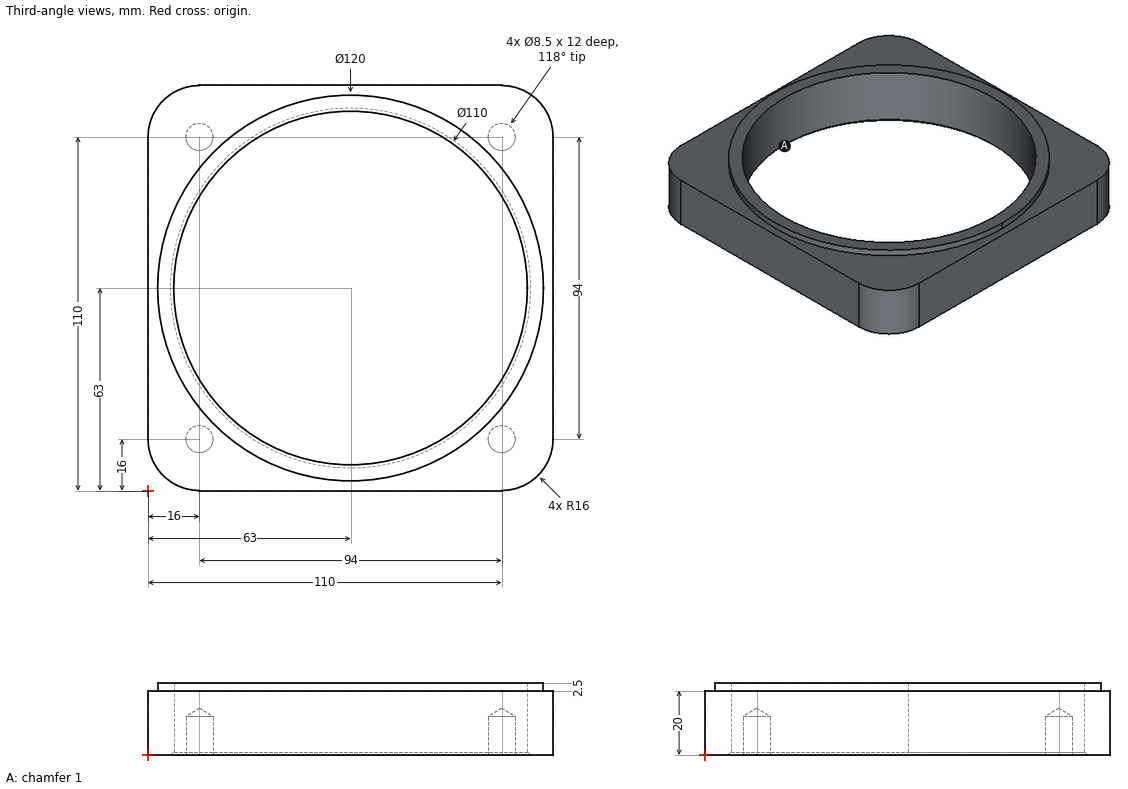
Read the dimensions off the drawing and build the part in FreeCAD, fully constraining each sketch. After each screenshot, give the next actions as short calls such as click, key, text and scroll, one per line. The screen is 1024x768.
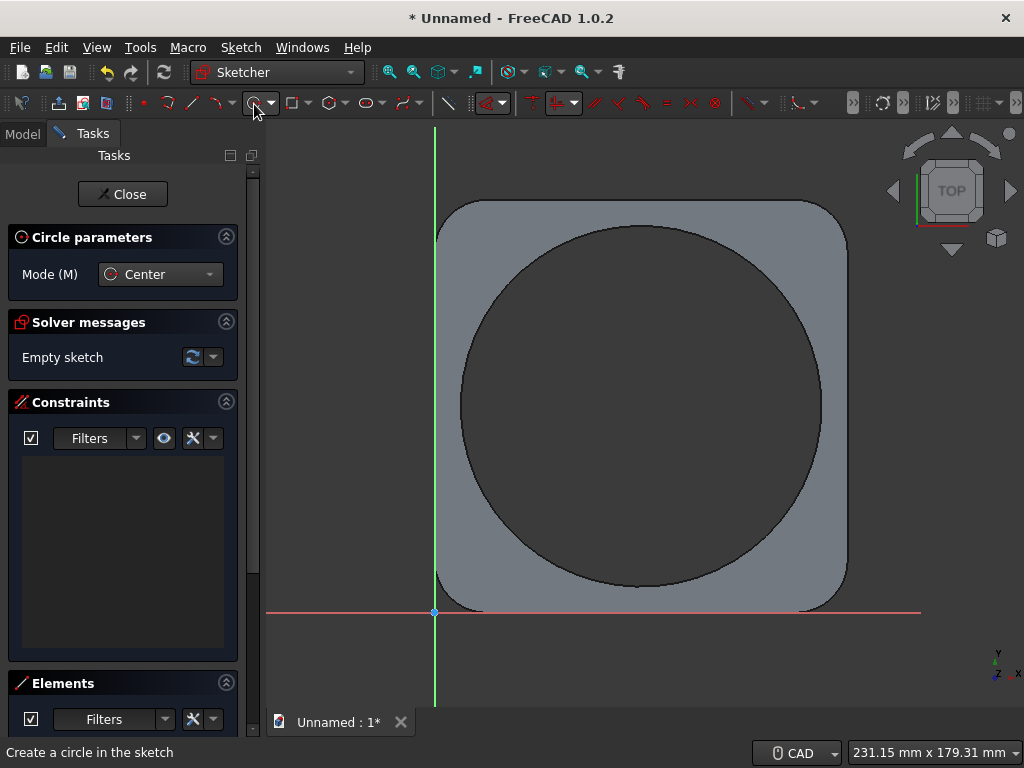
scroll(795, 252, up, 3)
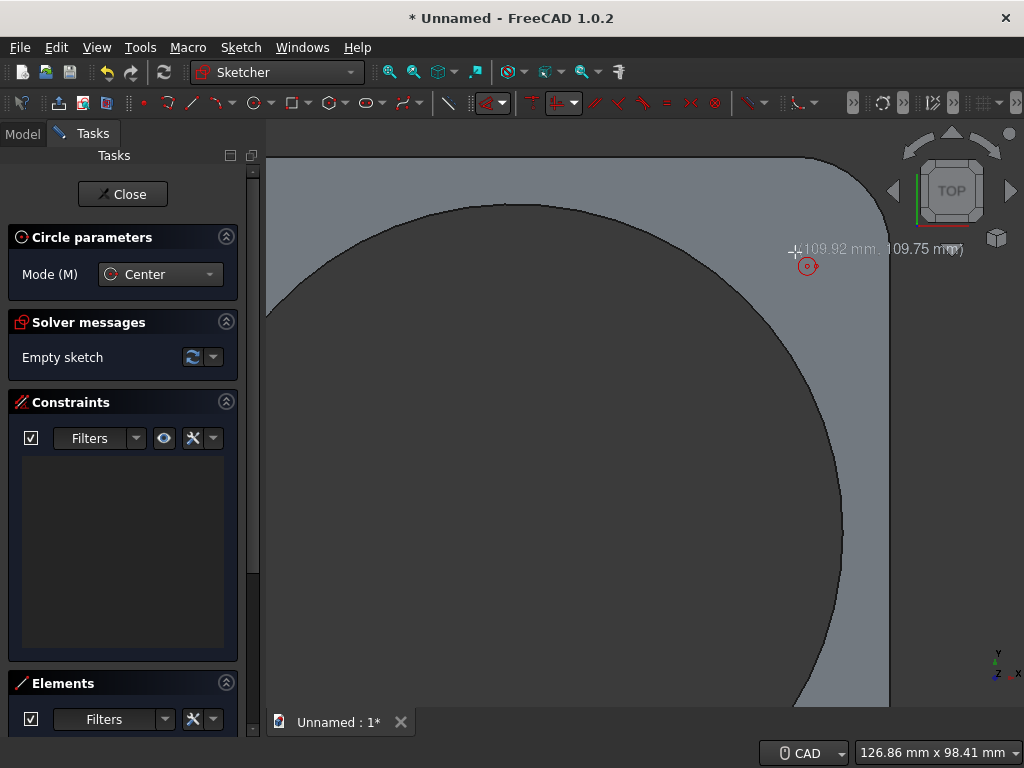
click(795, 252)
move(813, 234)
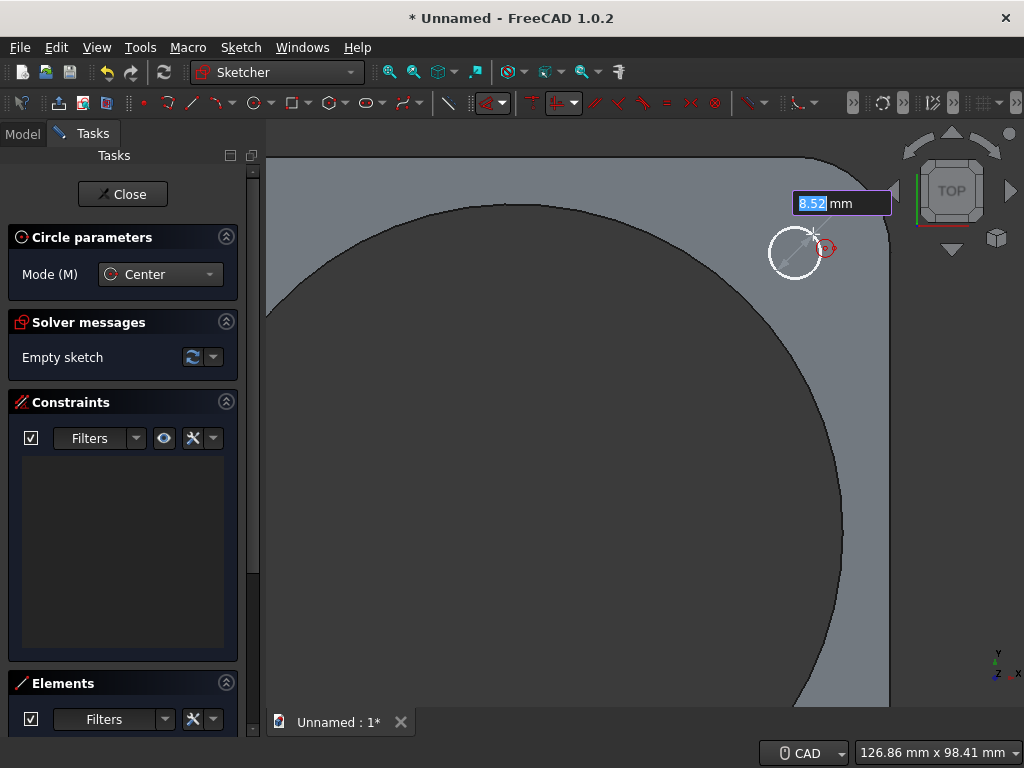
text(8.5)
key(Return)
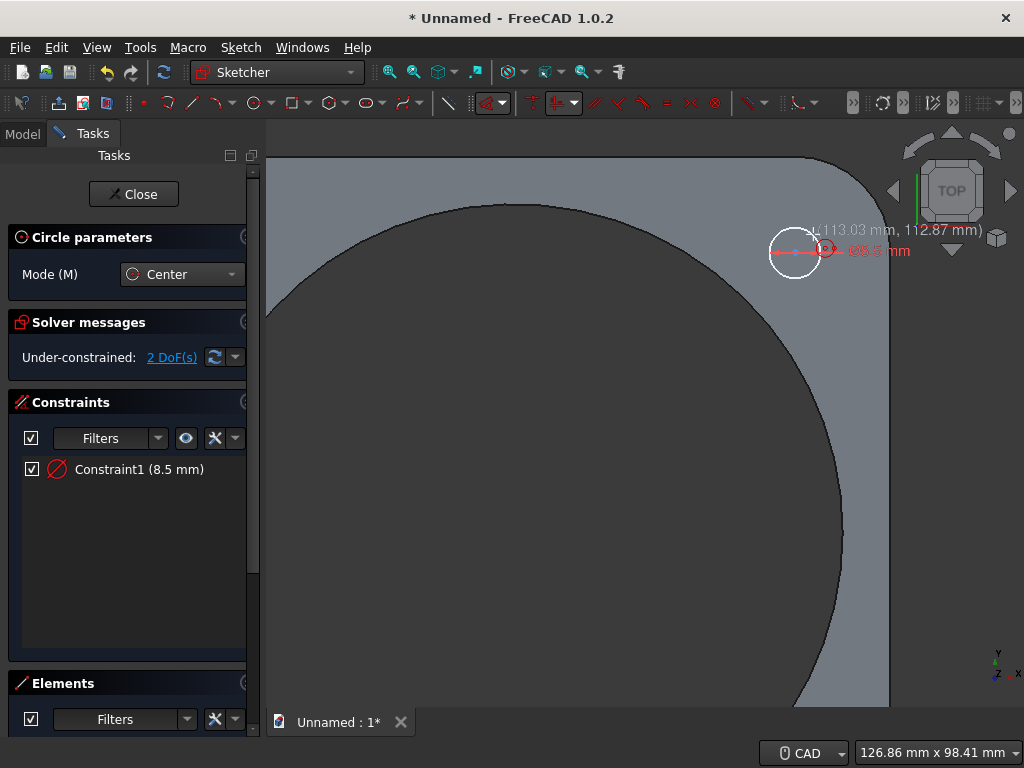
scroll(695, 224, down, 3)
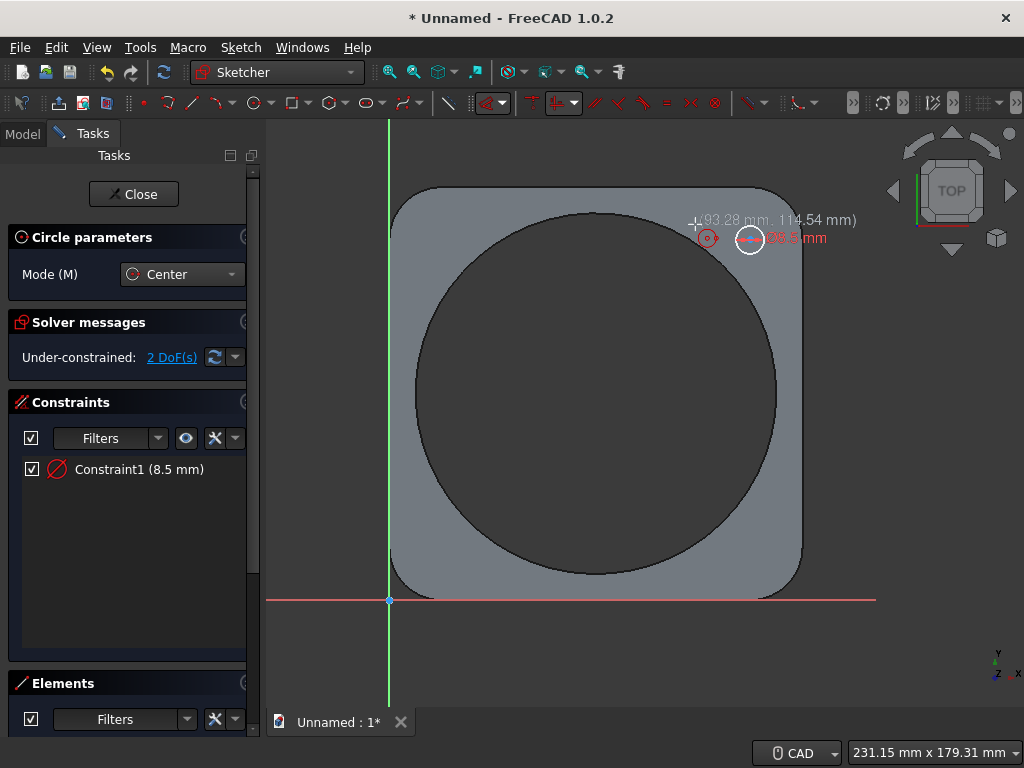
scroll(442, 240, up, 3)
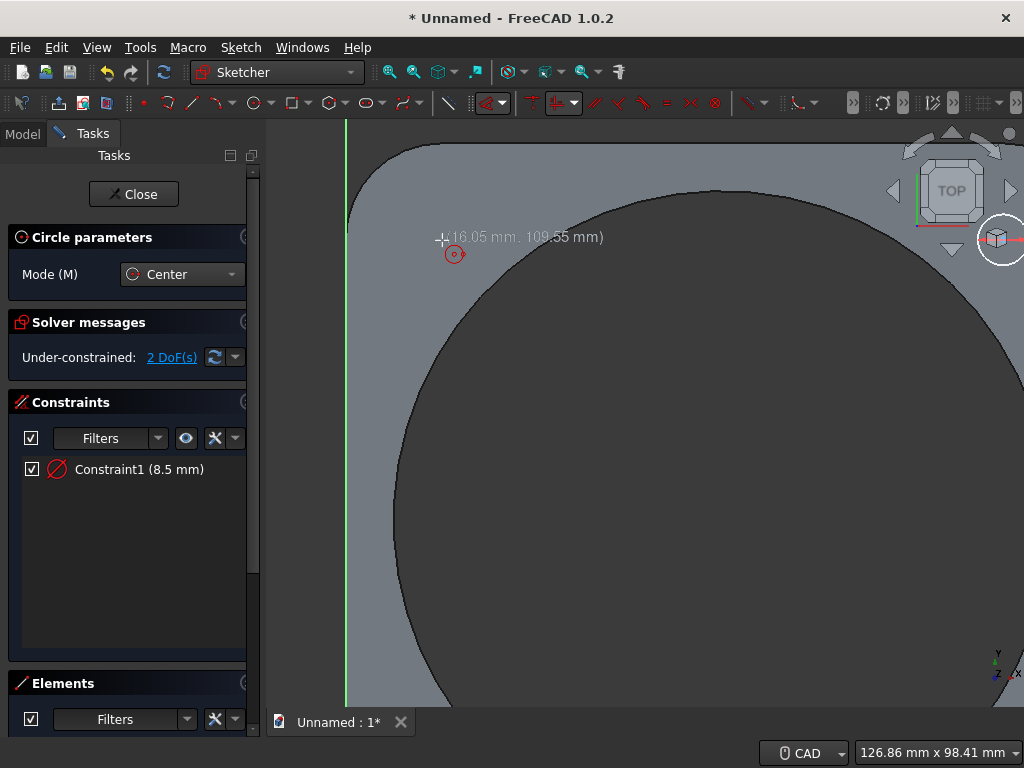
click(441, 239)
move(459, 221)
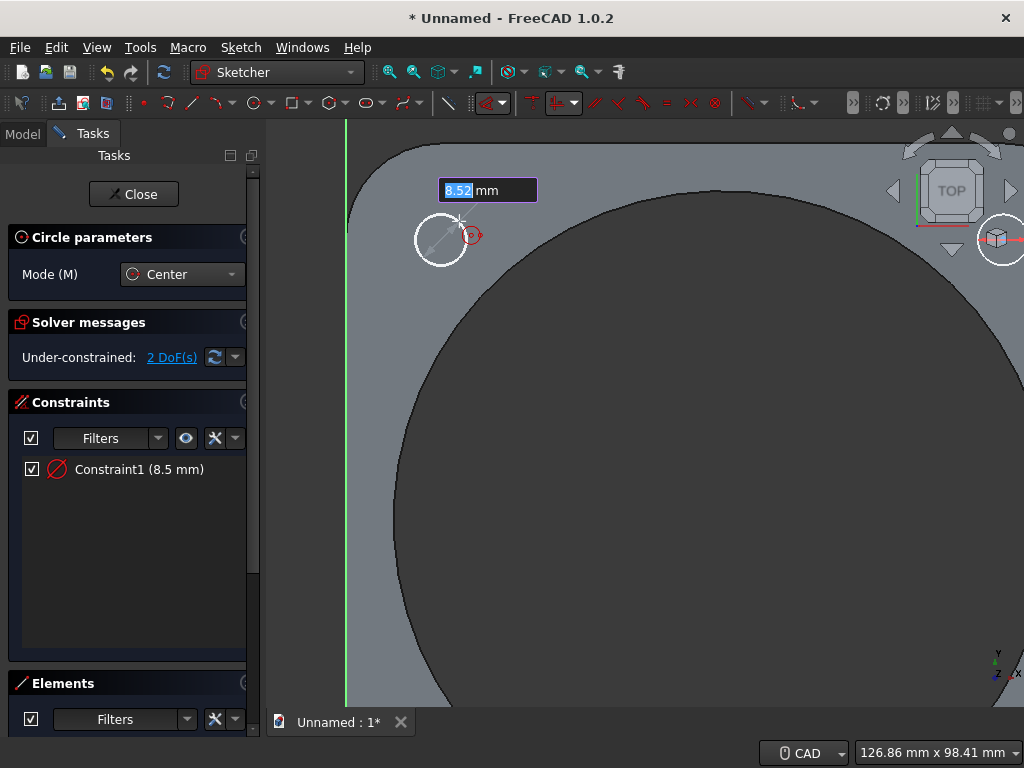
text(8.5)
key(Return)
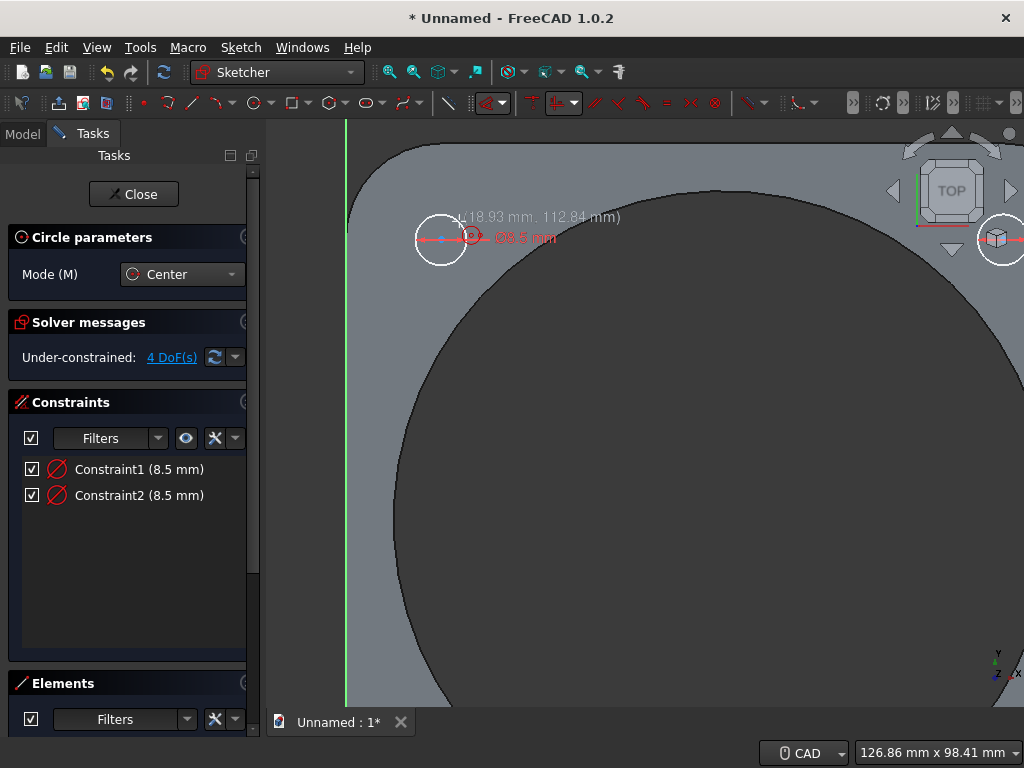
scroll(442, 240, down, 3)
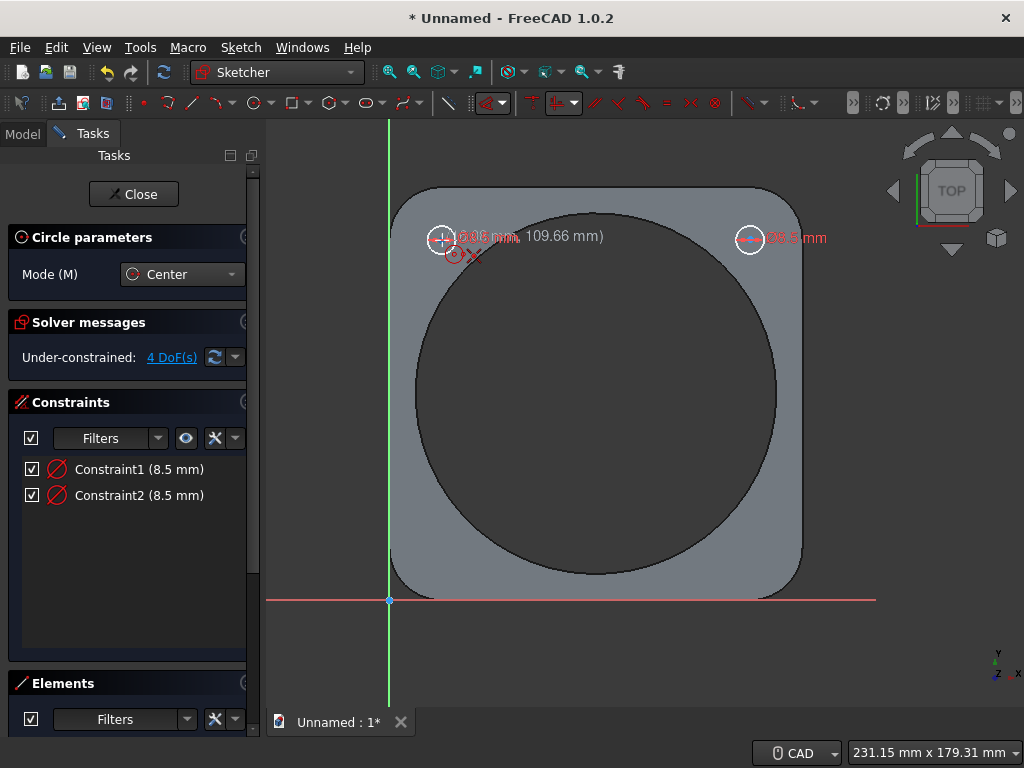
scroll(442, 548, up, 3)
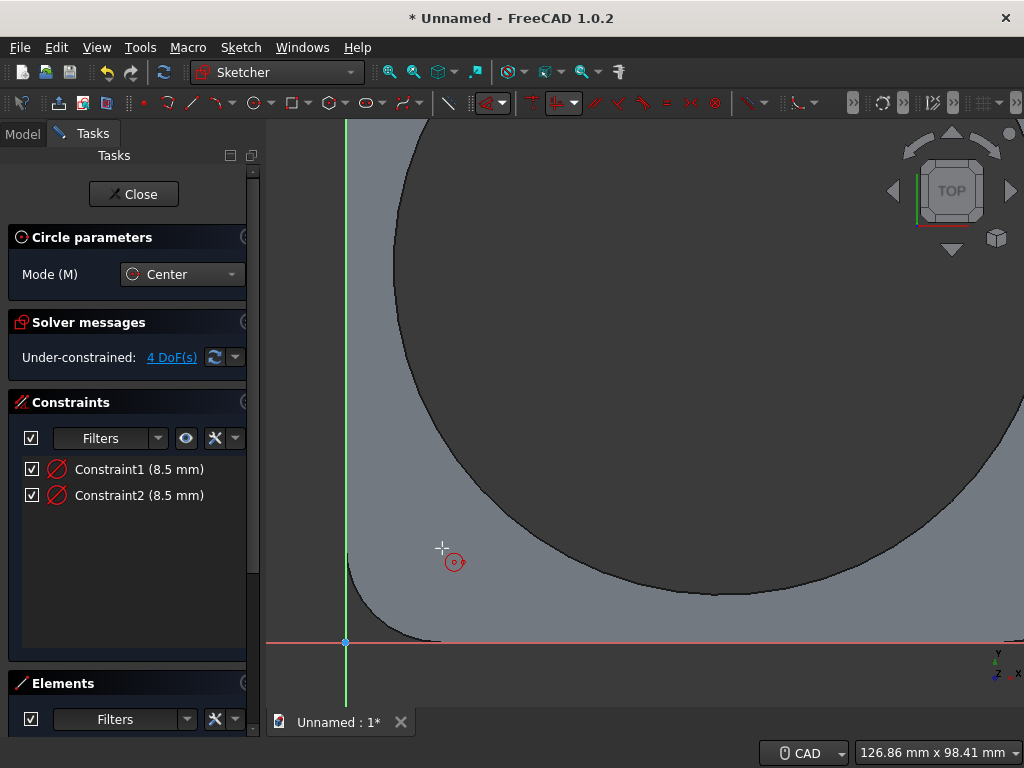
click(441, 547)
move(459, 529)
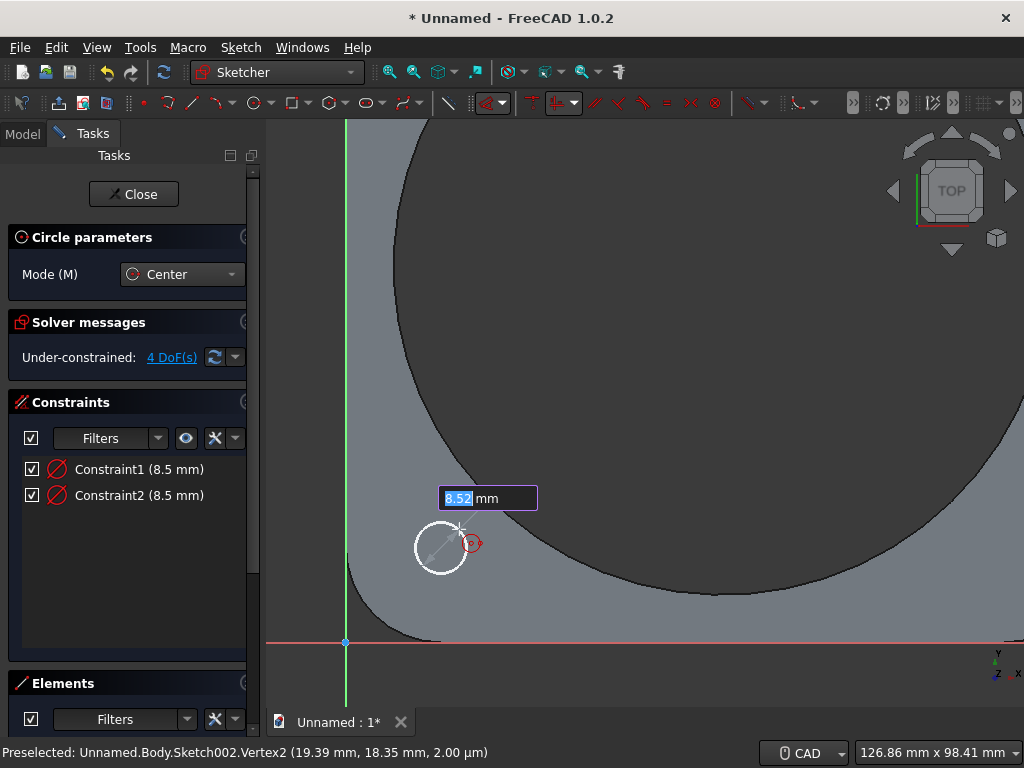
text(8.5)
key(Return)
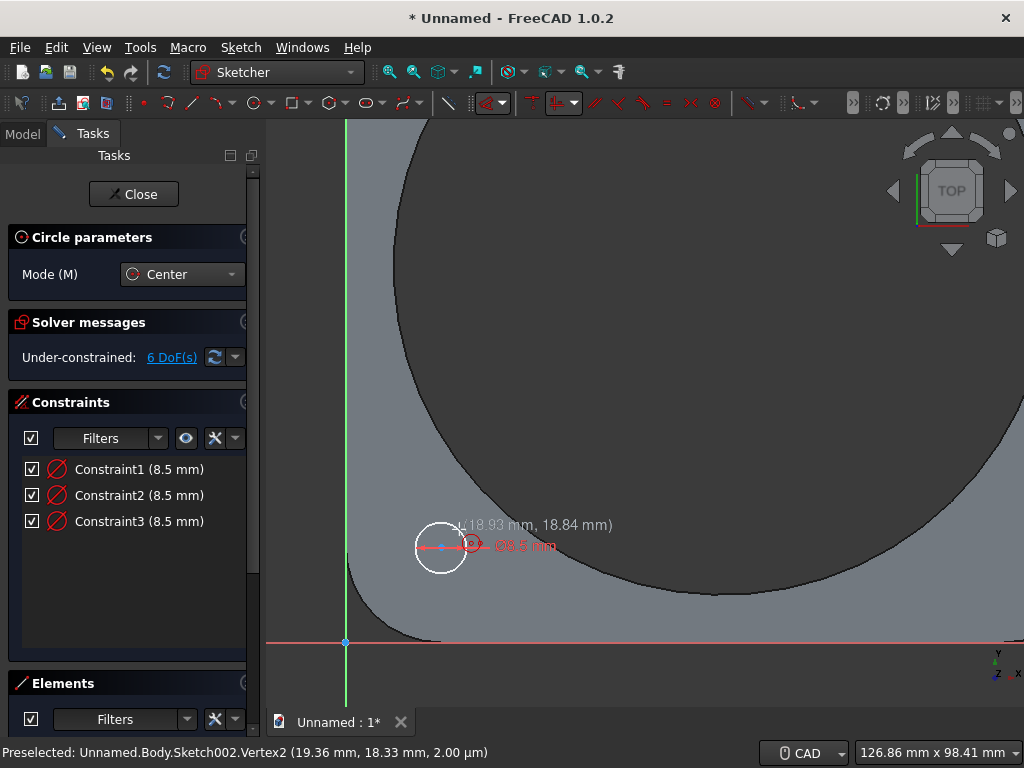
scroll(442, 549, down, 3)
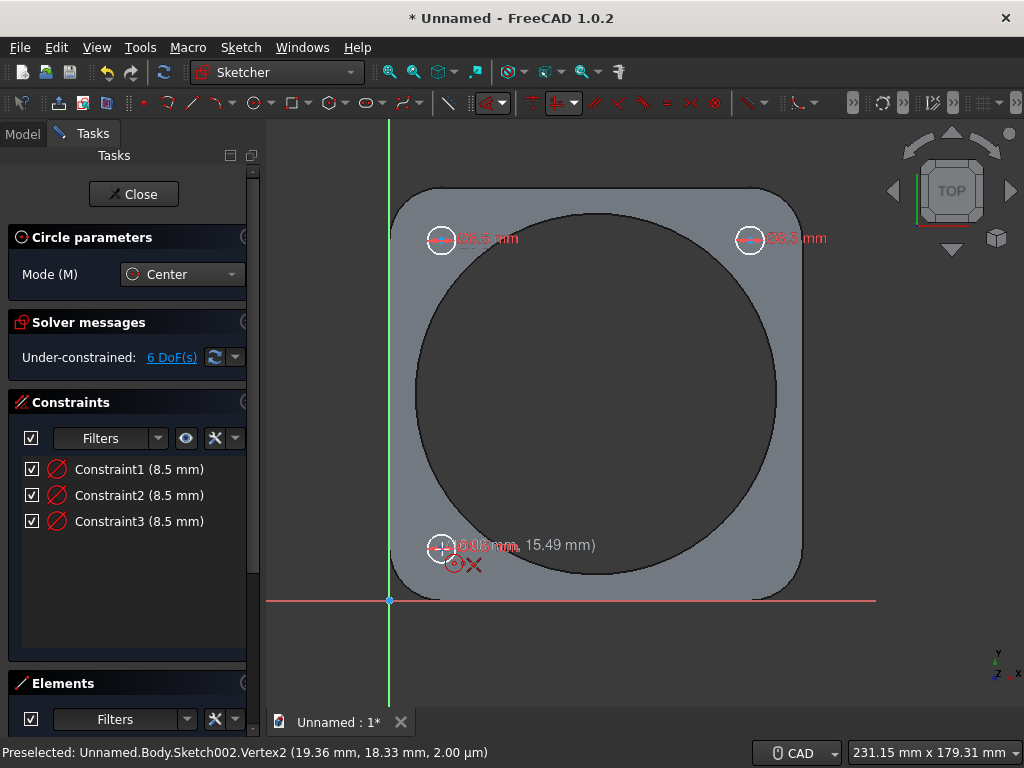
scroll(750, 548, up, 3)